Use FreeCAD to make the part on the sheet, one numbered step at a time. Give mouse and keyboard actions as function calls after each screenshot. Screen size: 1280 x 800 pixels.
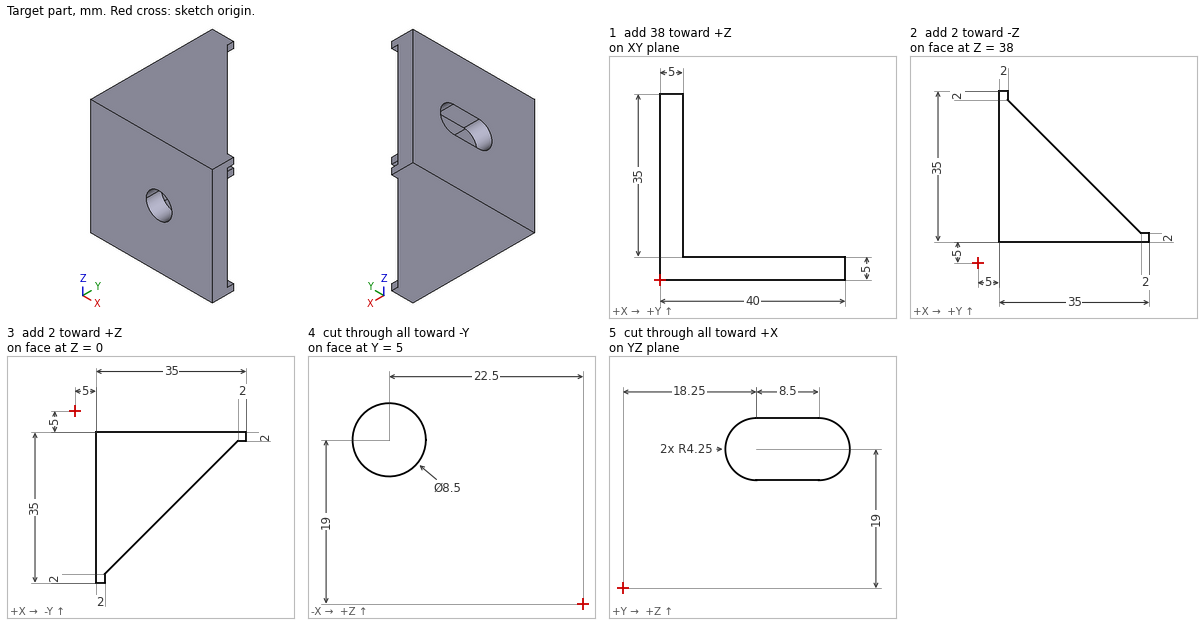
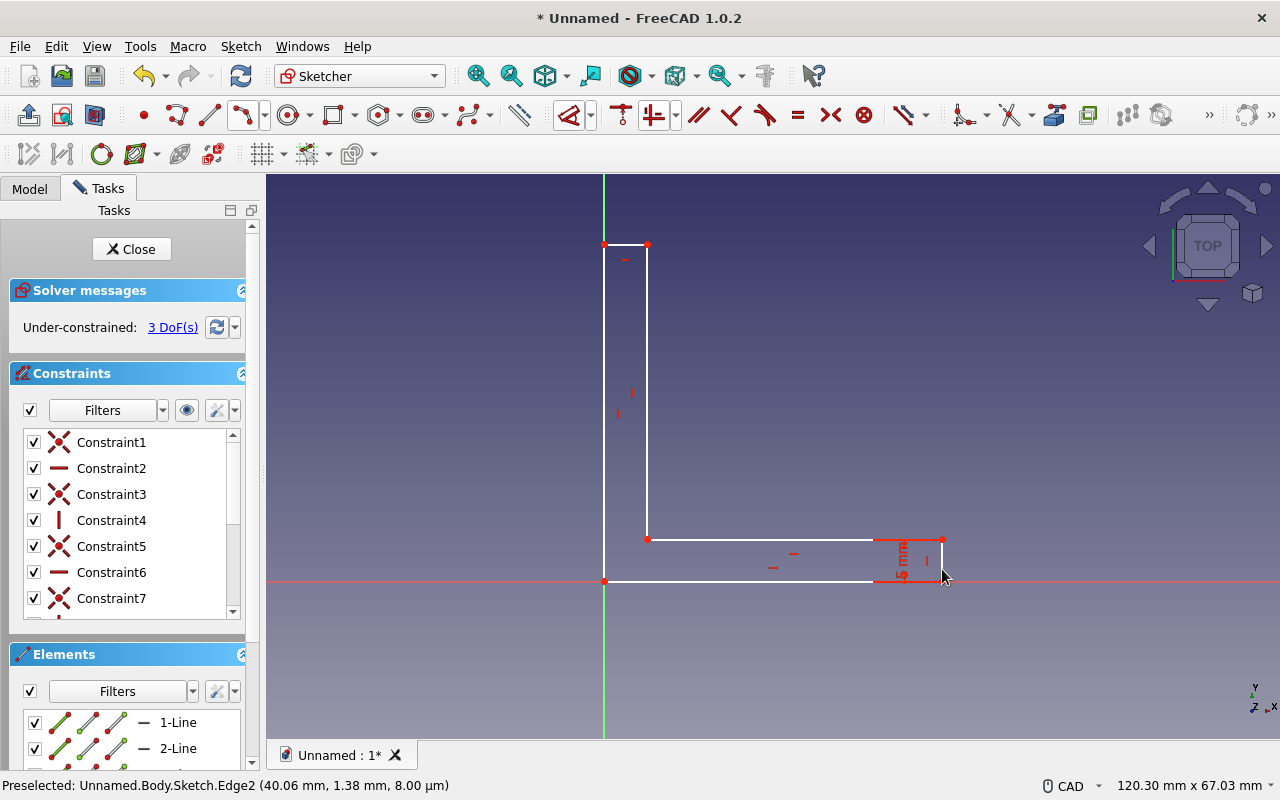
click(634, 245)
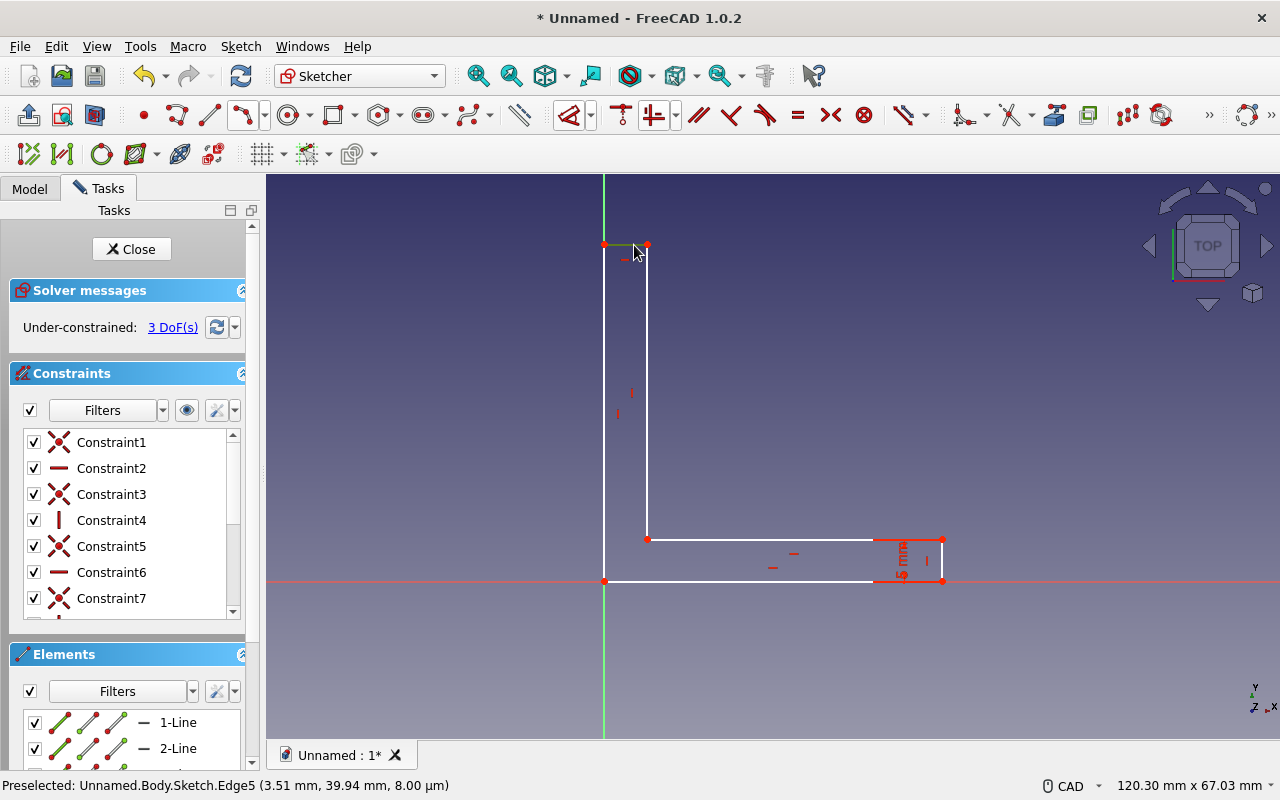
click(590, 116)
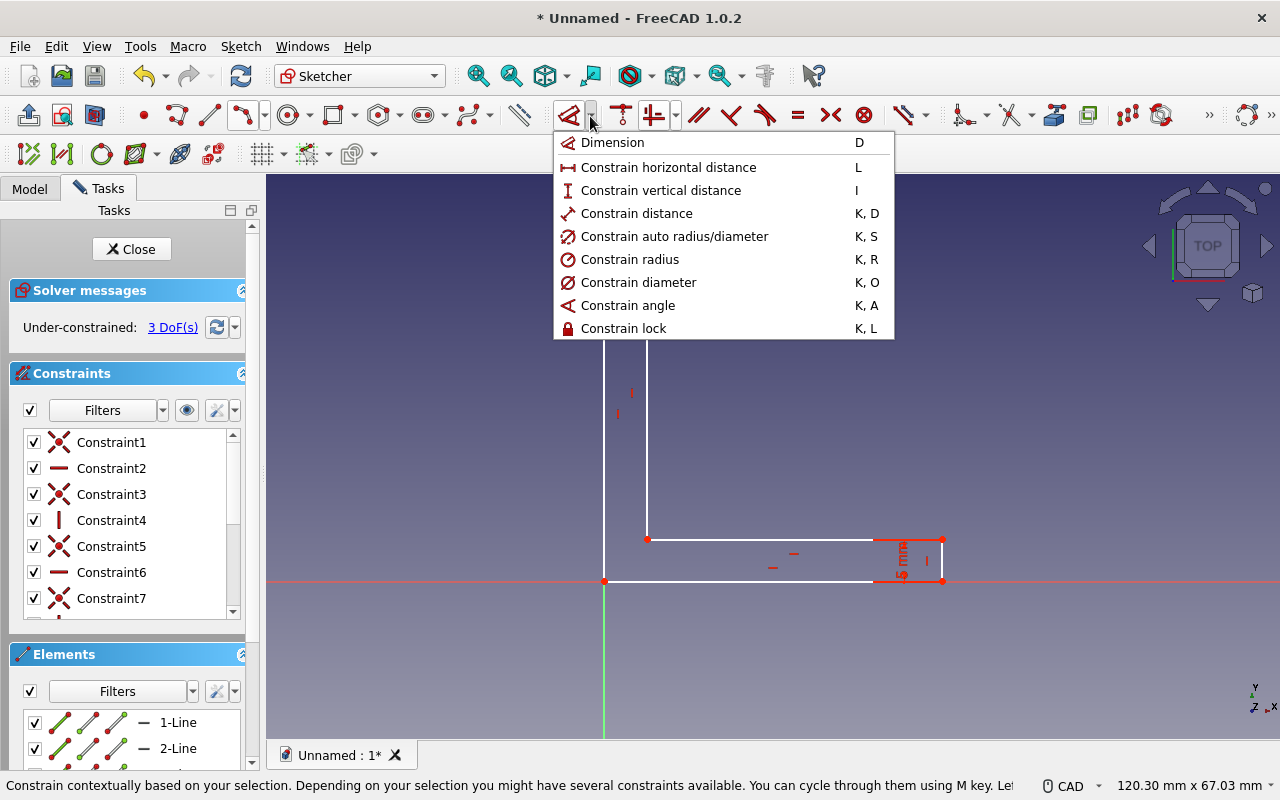
click(724, 168)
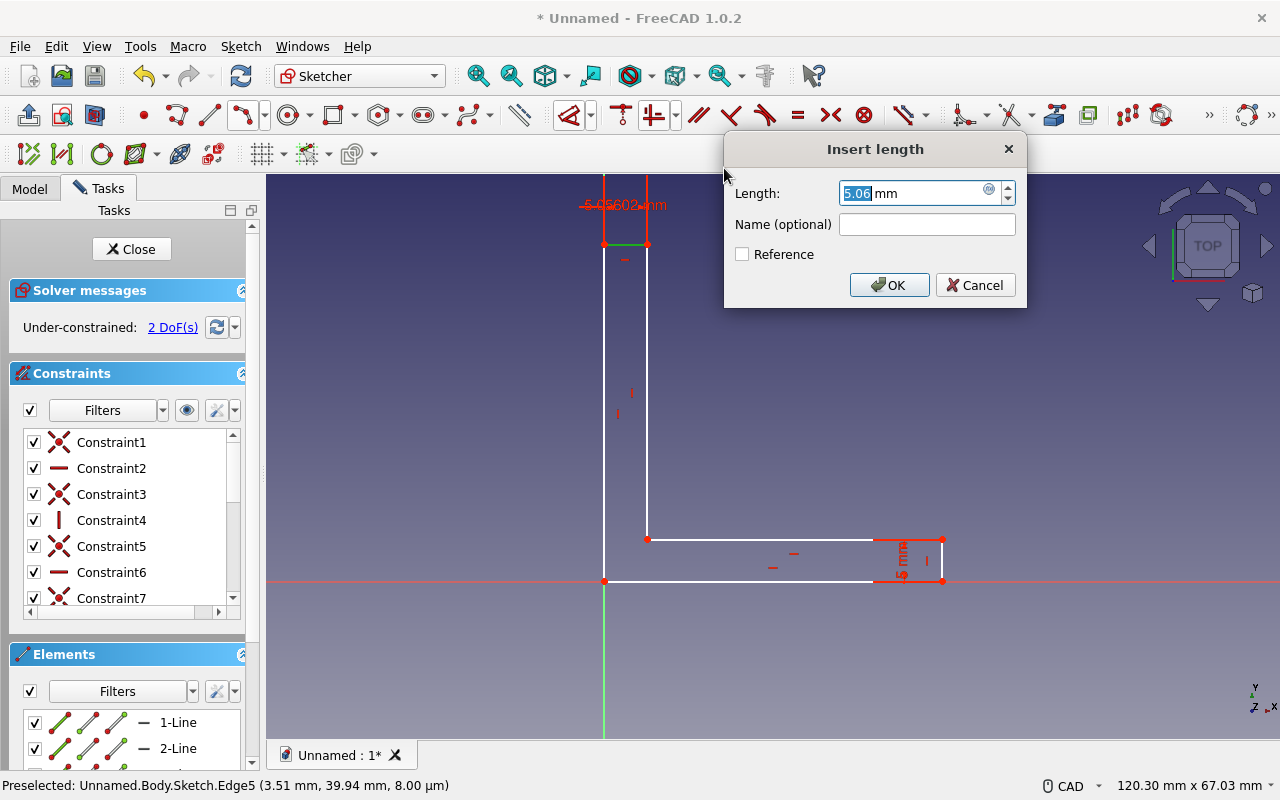
text(5)
key(Return)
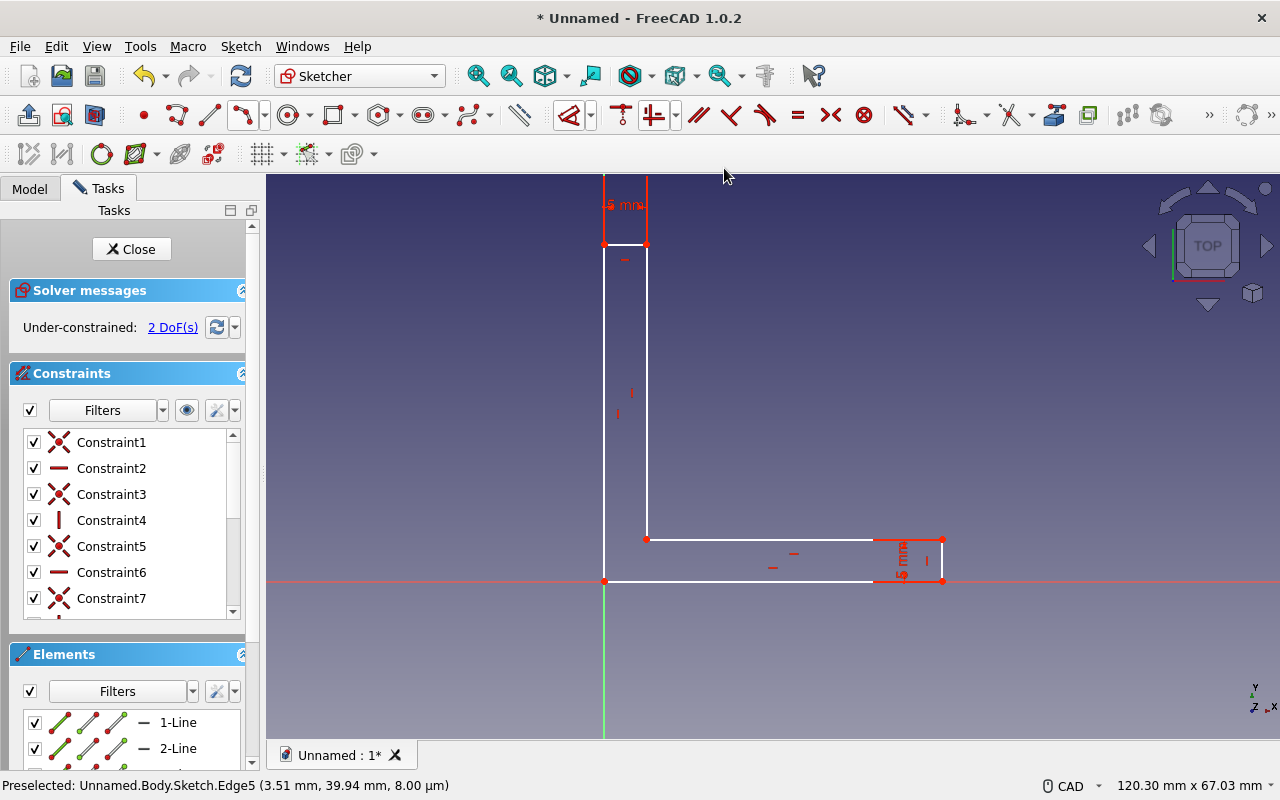
click(706, 582)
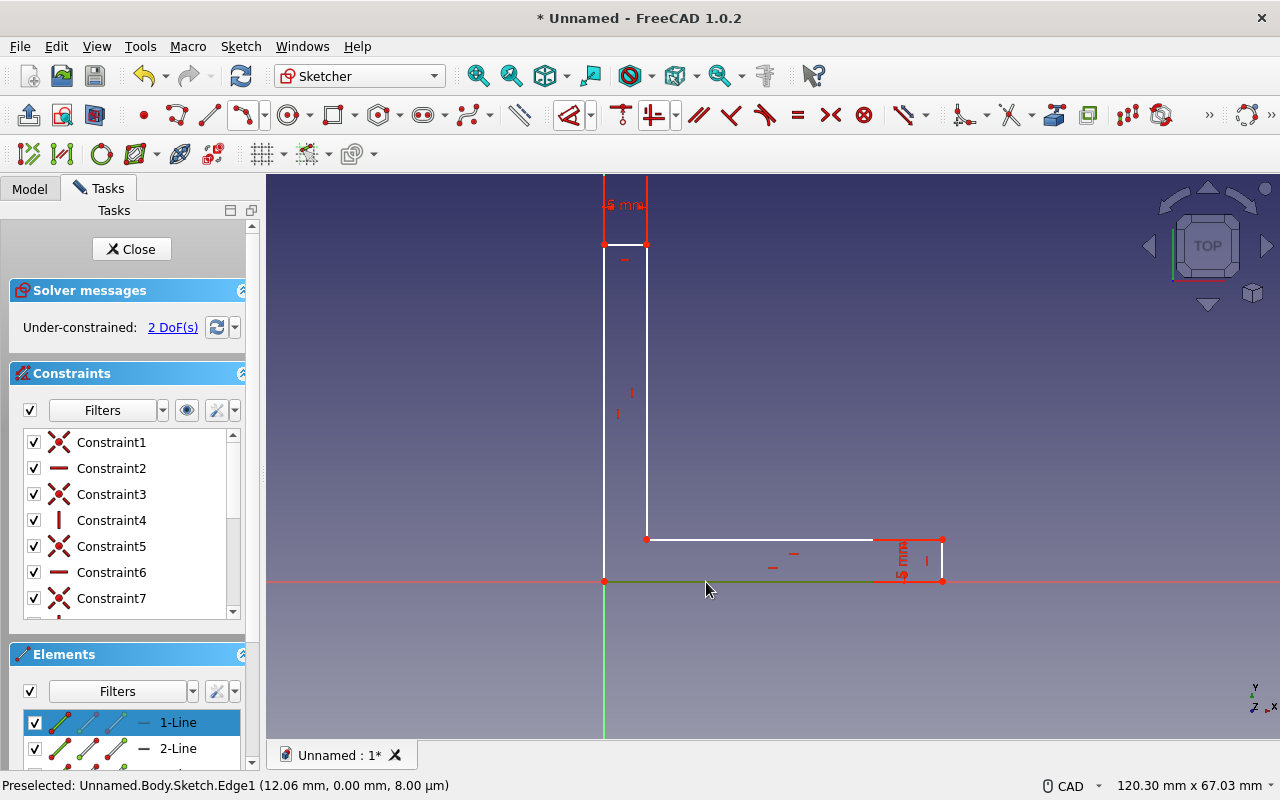
key(l)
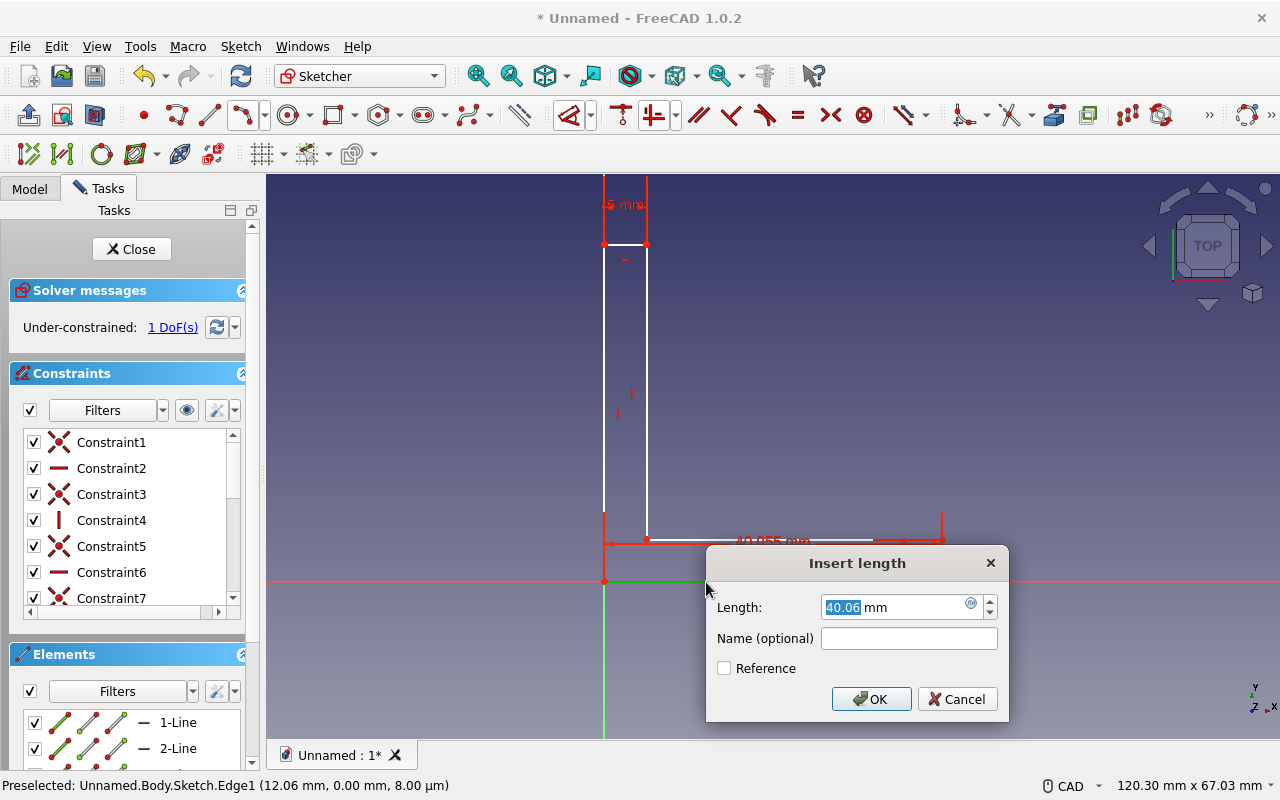
text(40)
key(Return)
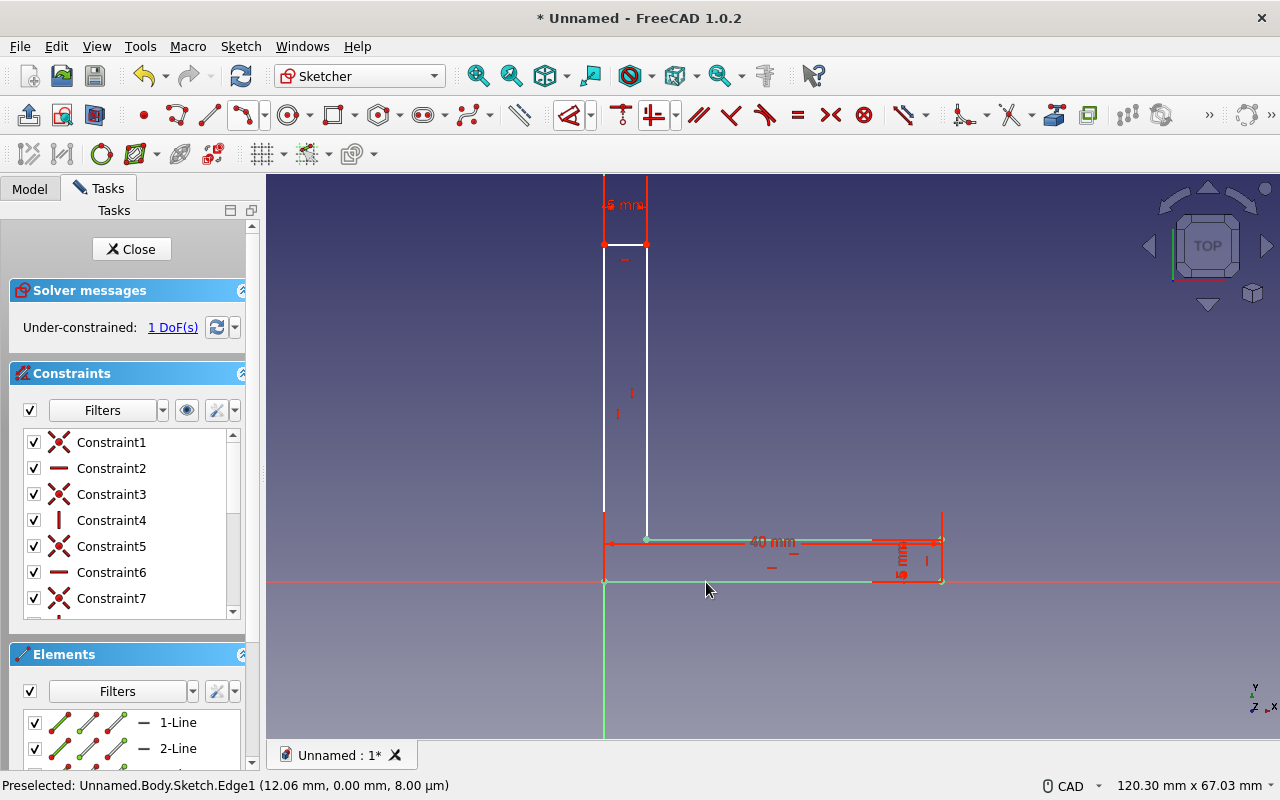
click(647, 451)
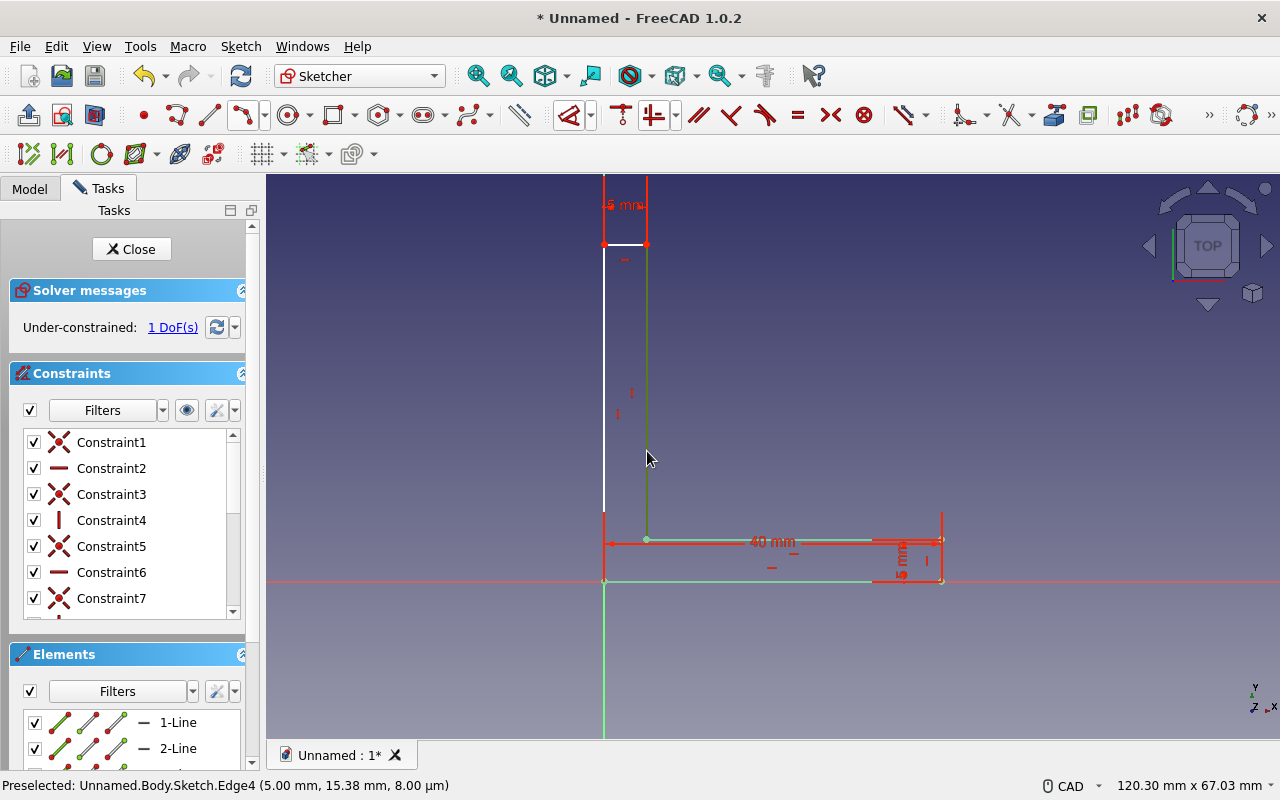
click(590, 116)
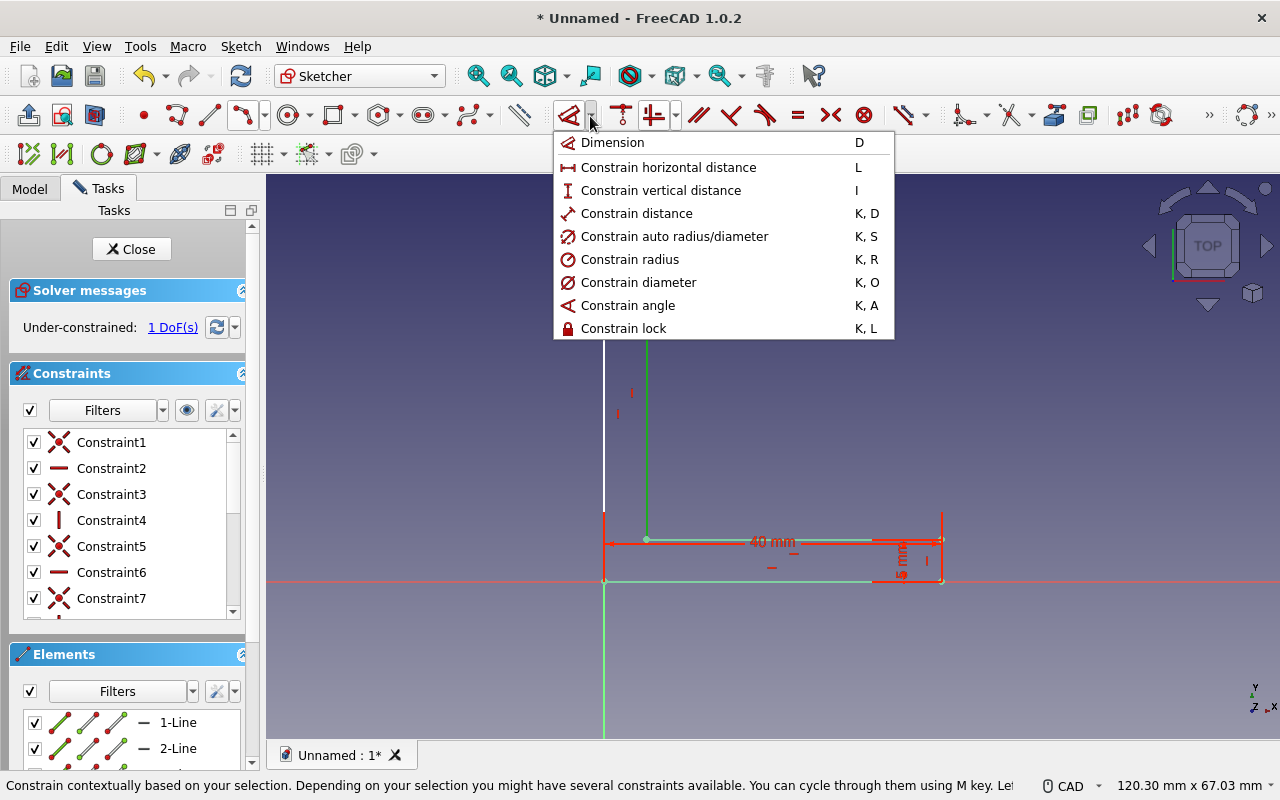
click(724, 190)